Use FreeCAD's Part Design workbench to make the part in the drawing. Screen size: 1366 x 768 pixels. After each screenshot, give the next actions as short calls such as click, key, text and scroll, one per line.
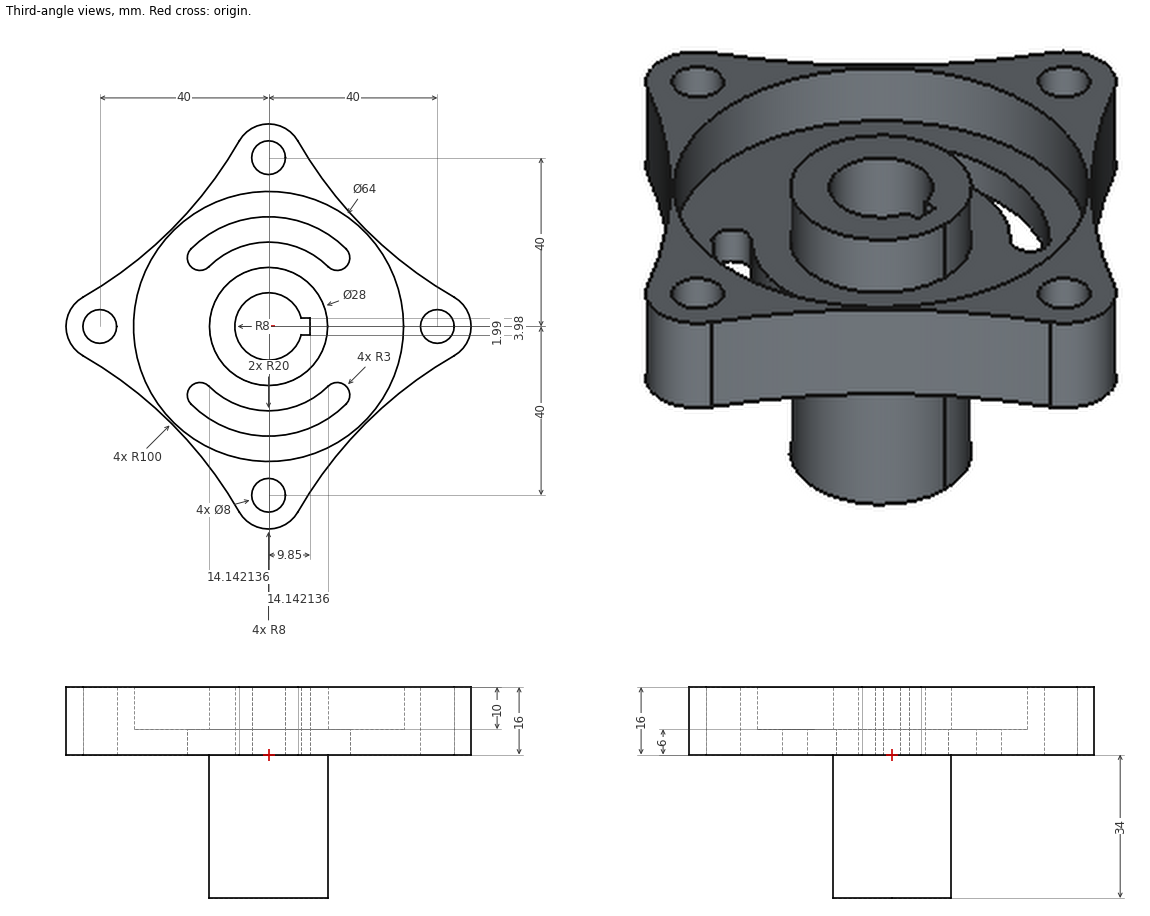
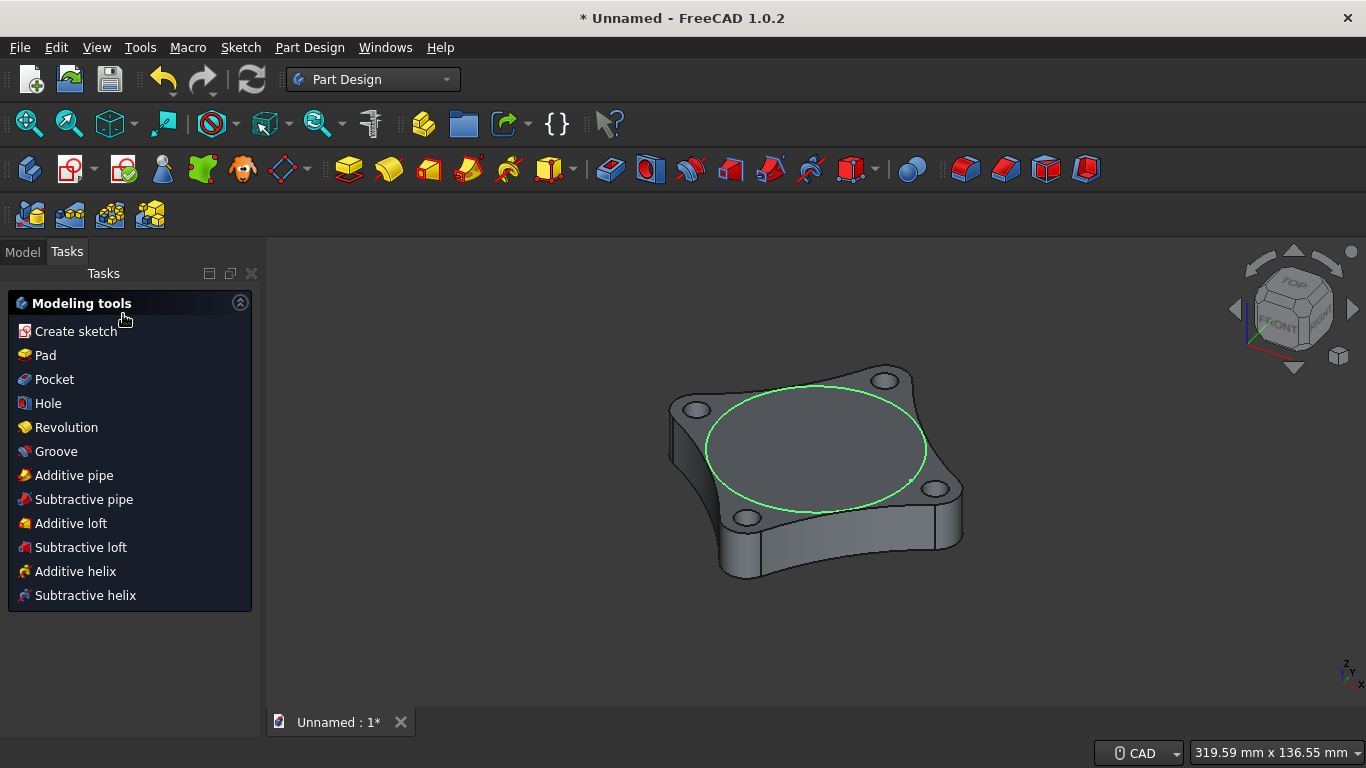
click(612, 170)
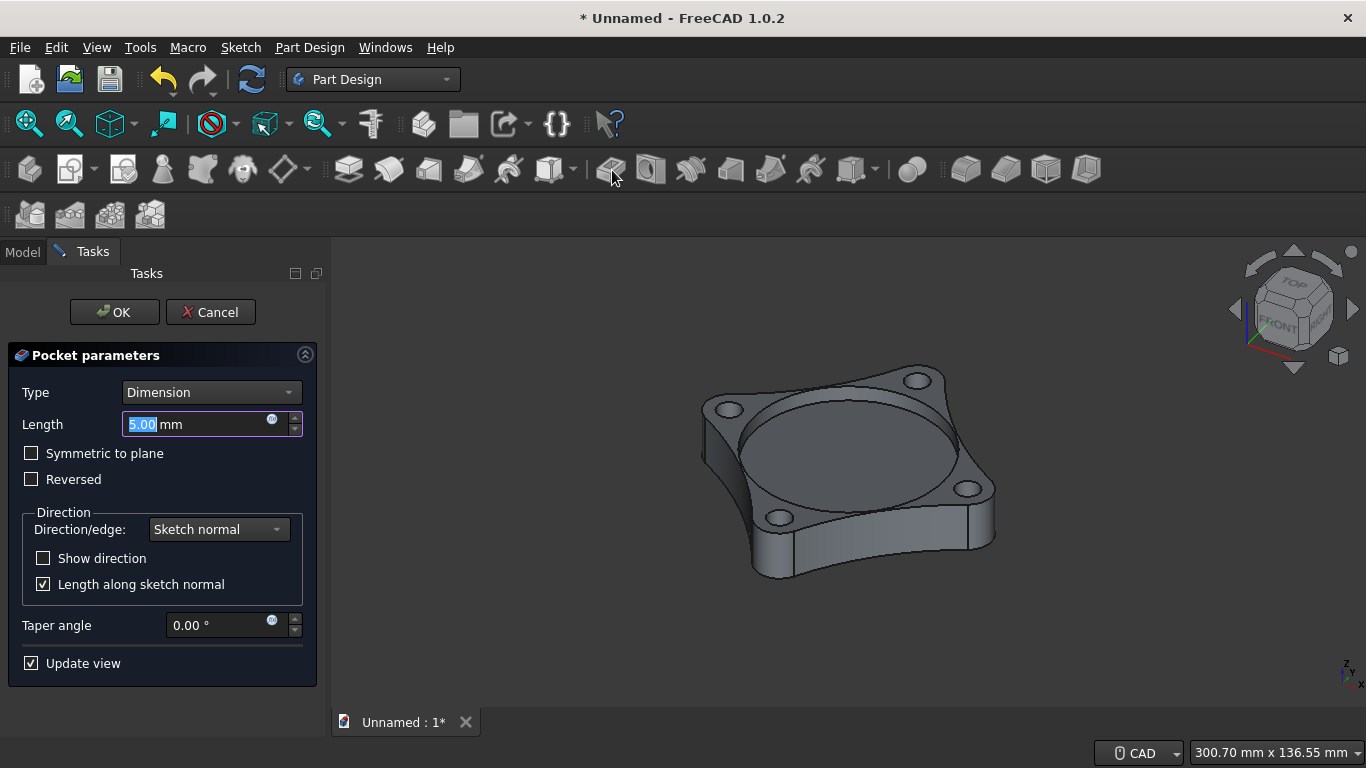
text(10)
key(Tab)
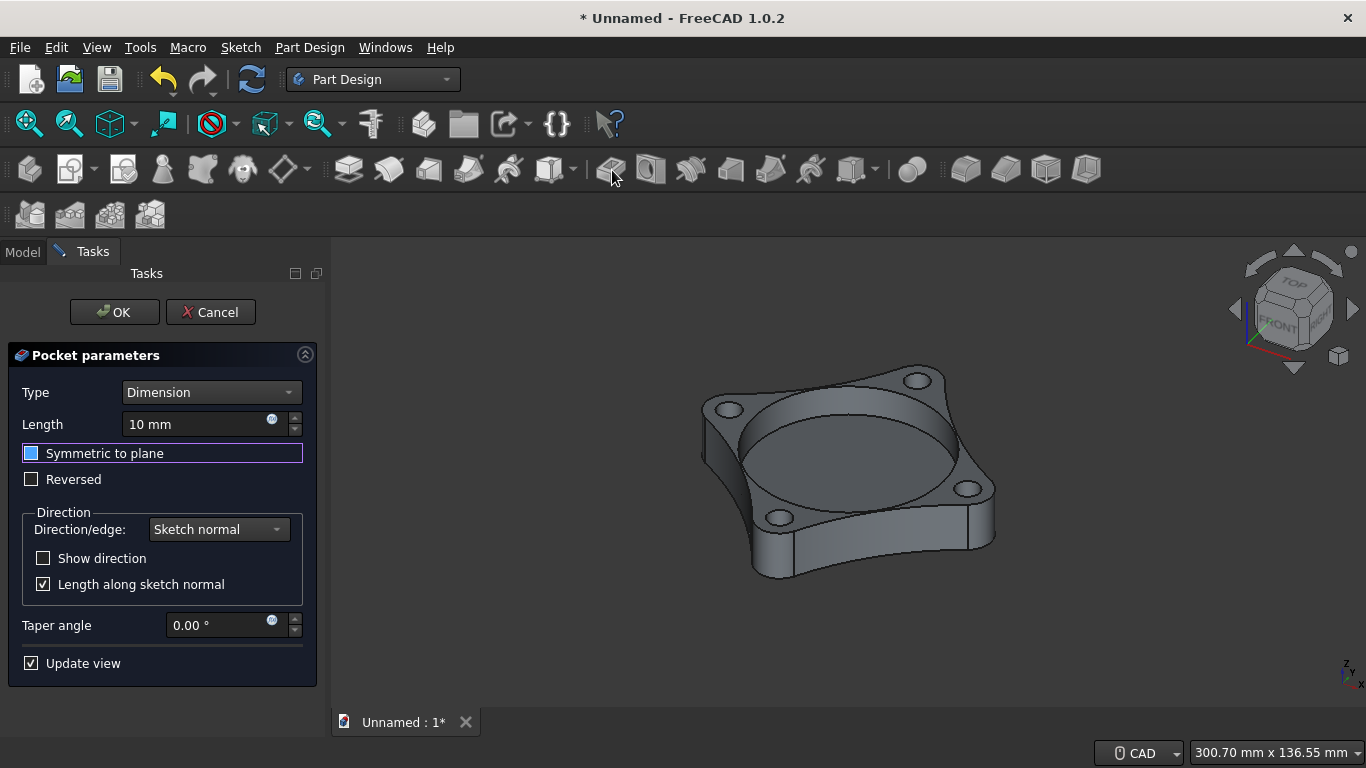
click(115, 312)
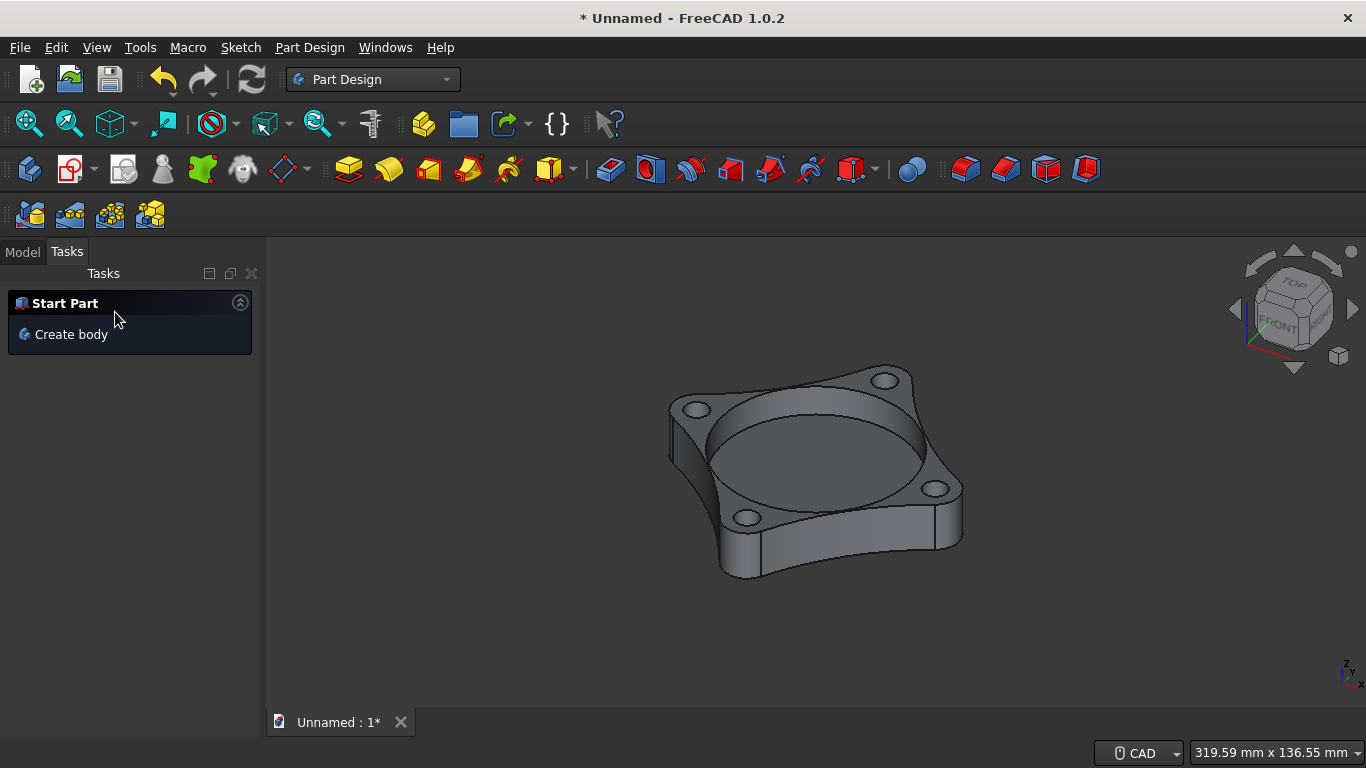
click(816, 477)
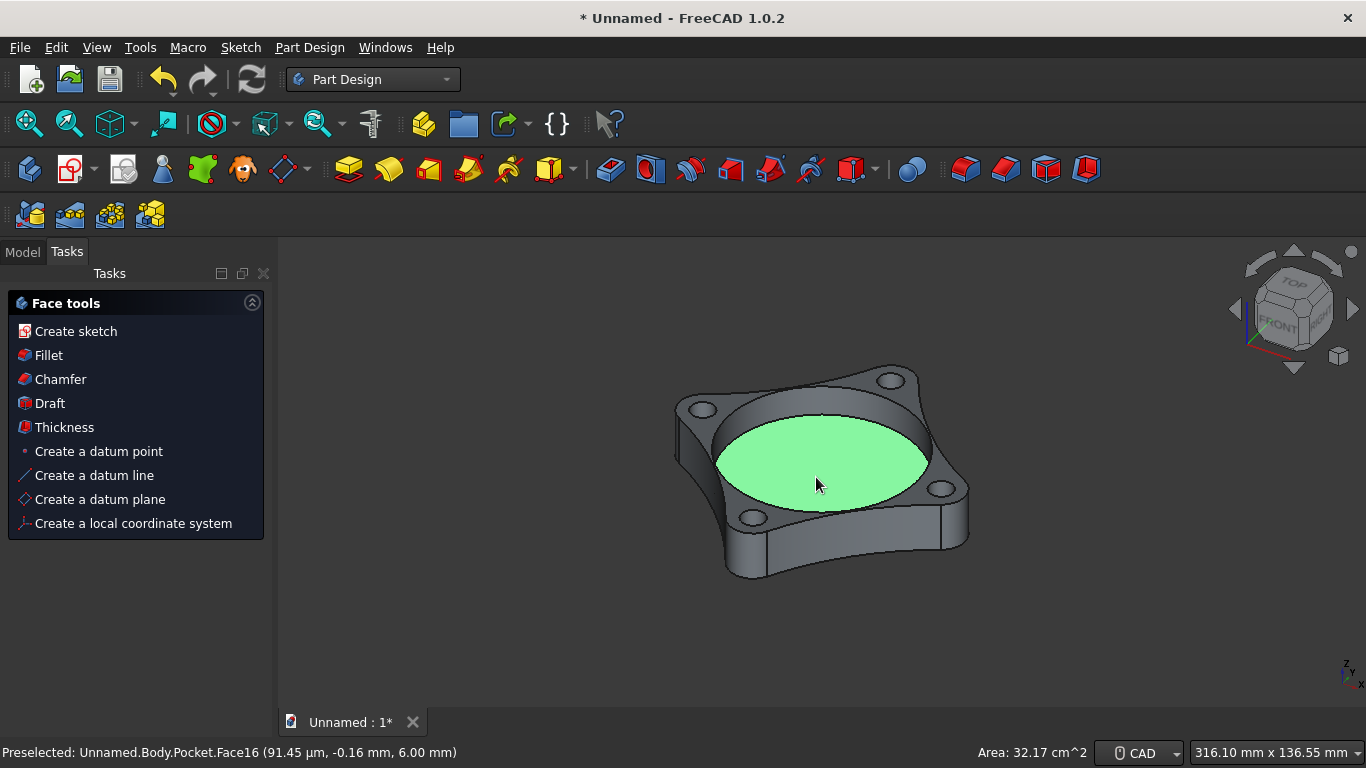
click(70, 170)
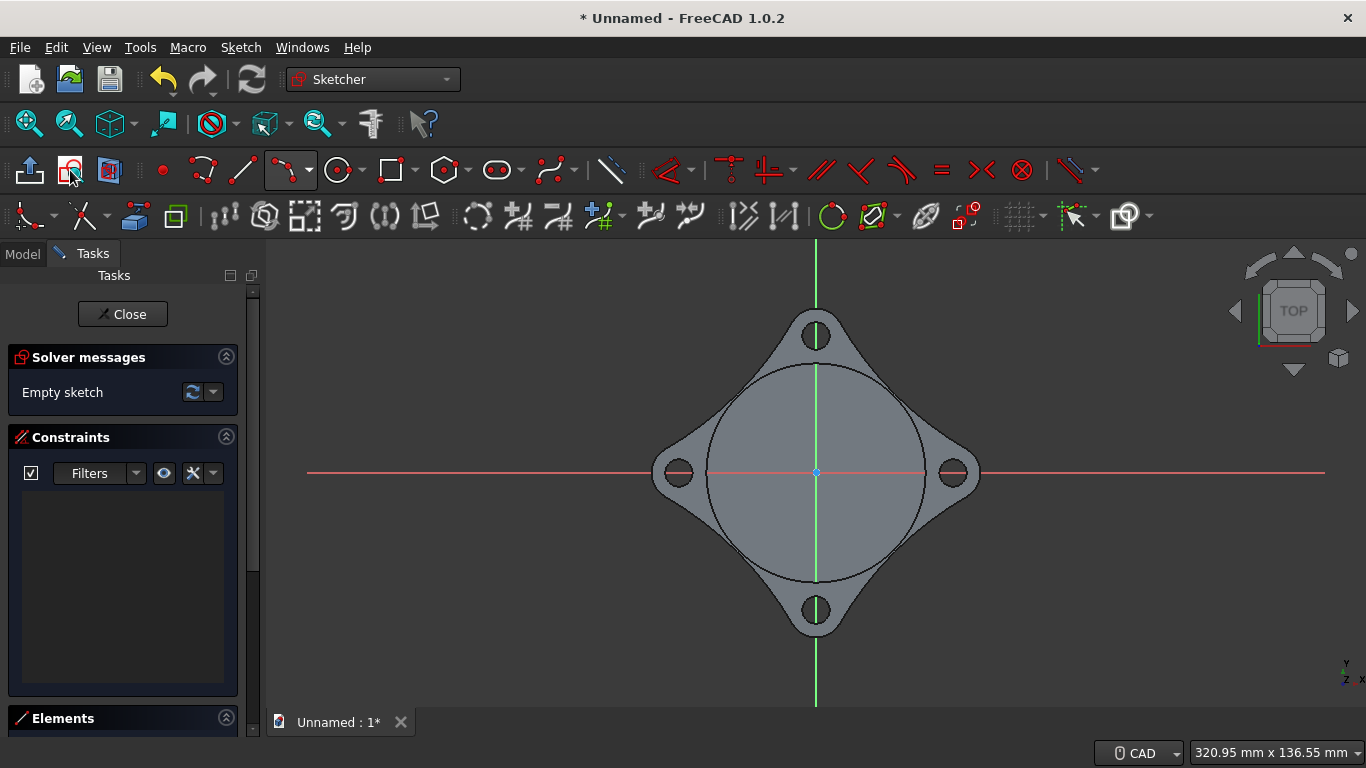
click(110, 170)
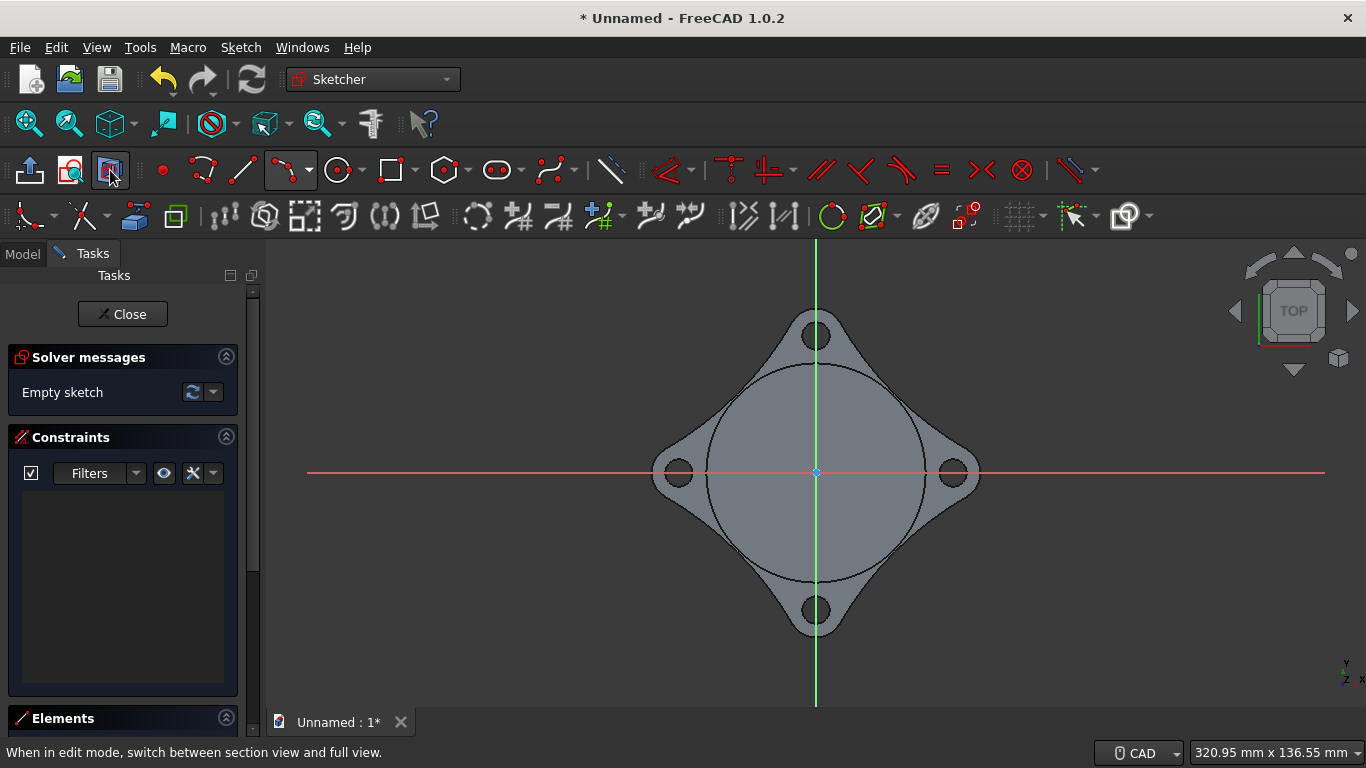
scroll(955, 473, up, 2)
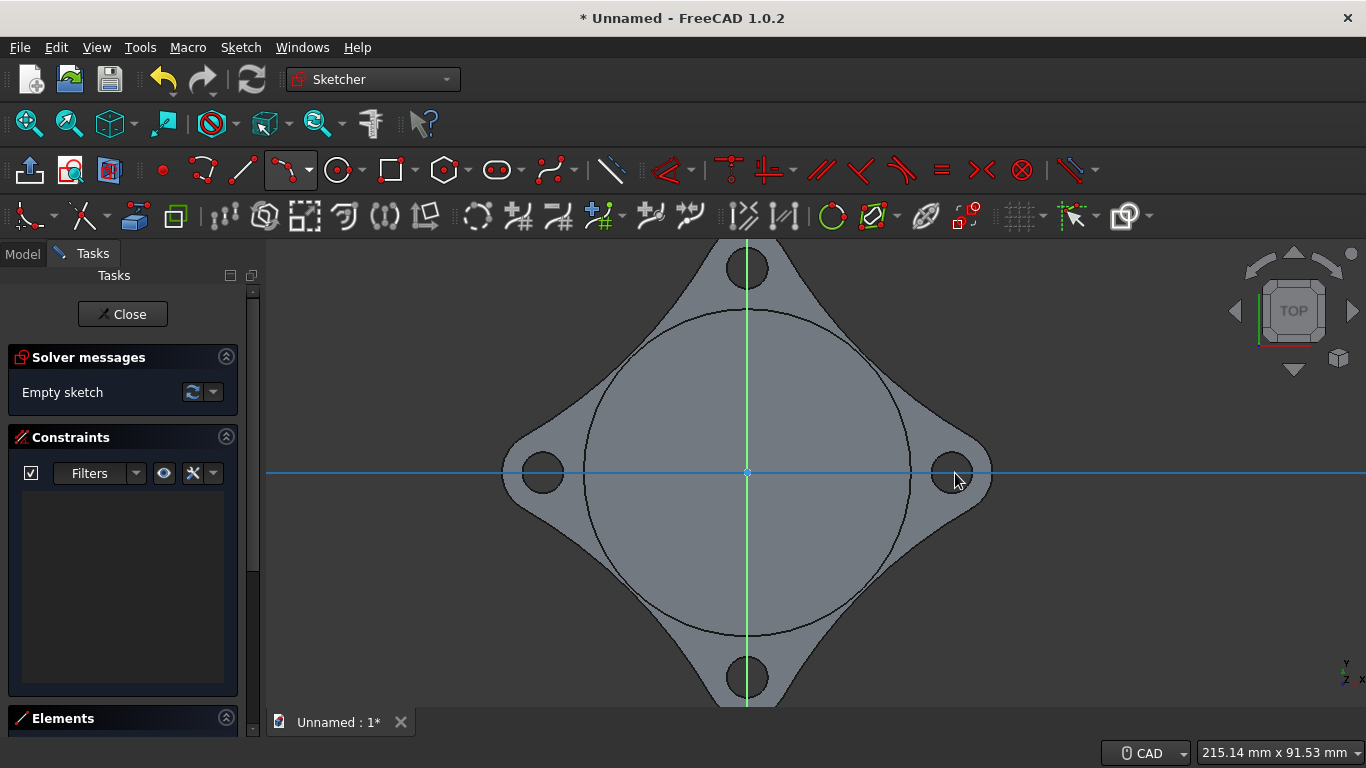
click(284, 170)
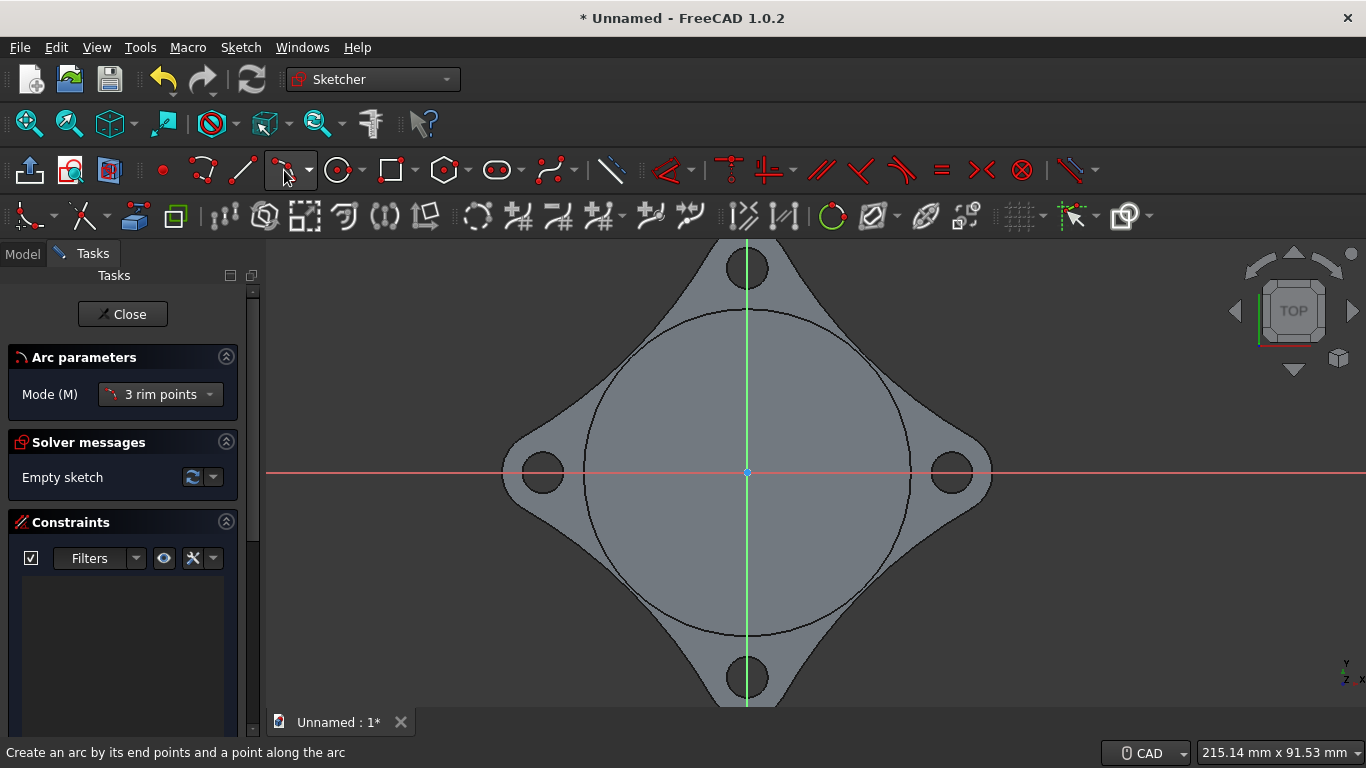
click(820, 545)
click(675, 545)
click(731, 574)